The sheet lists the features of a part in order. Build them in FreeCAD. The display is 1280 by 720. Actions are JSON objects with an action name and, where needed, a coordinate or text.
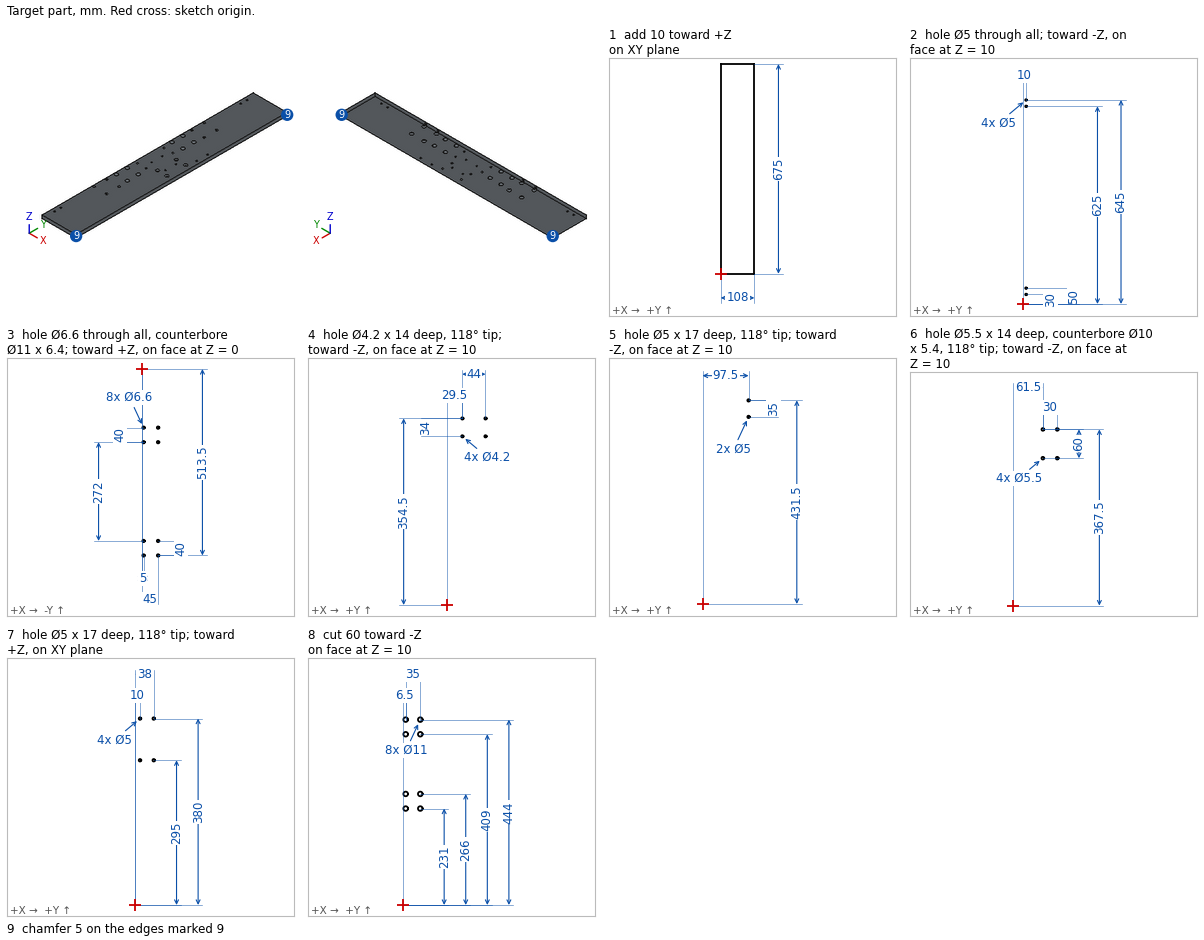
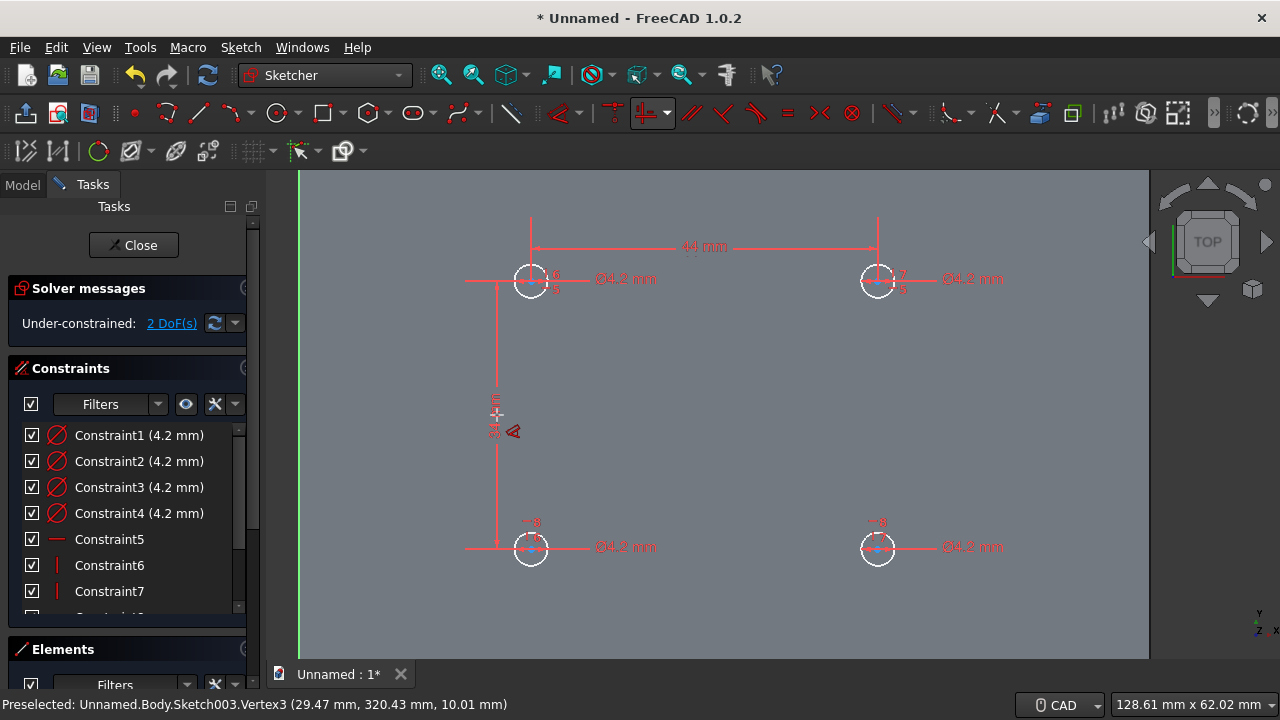
{"action": "left_click", "coordinate": [531, 281]}
{"action": "left_click", "coordinate": [415, 247]}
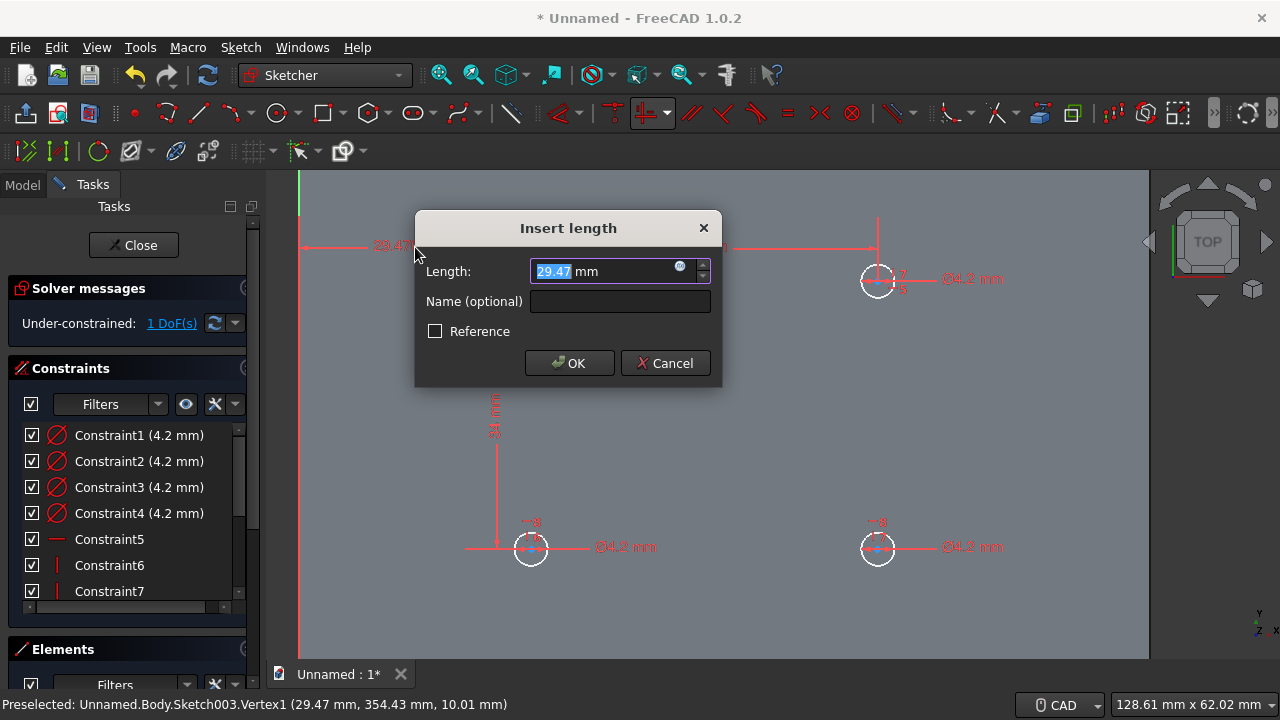
{"action": "type", "text": "29.5"}
{"action": "key", "text": "Return"}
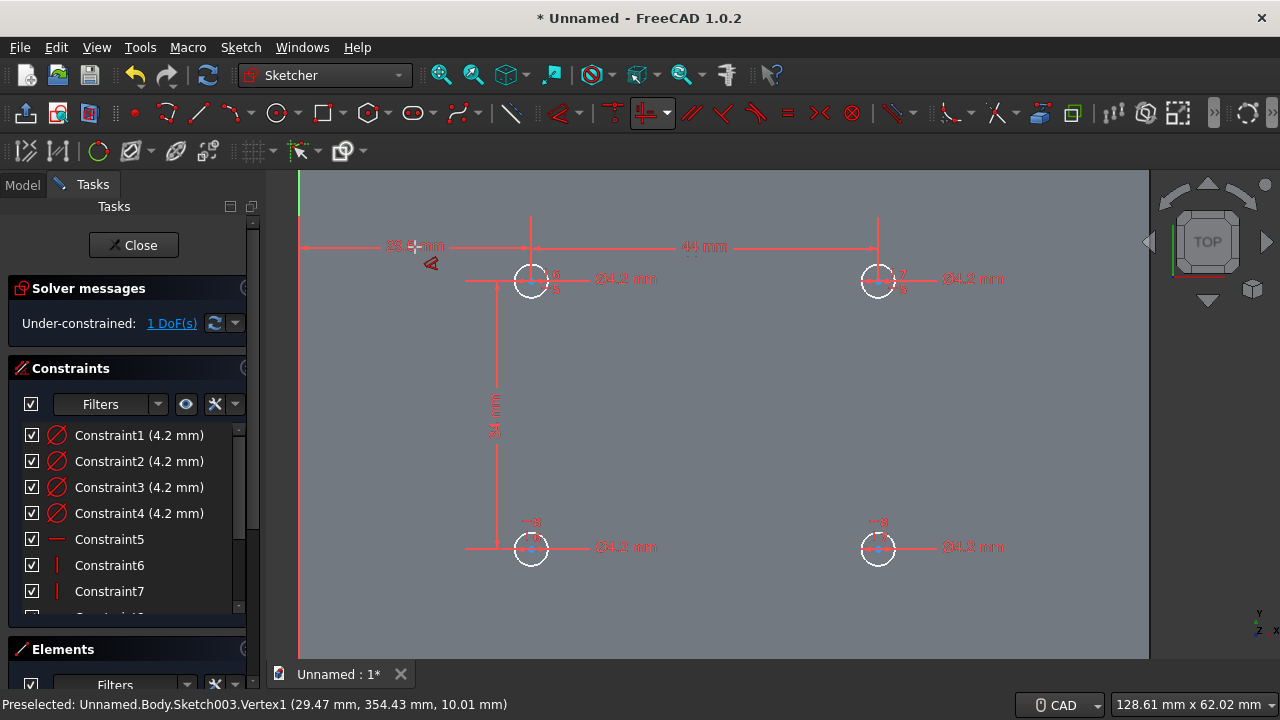
{"action": "left_click", "coordinate": [531, 281]}
{"action": "left_click", "coordinate": [565, 456]}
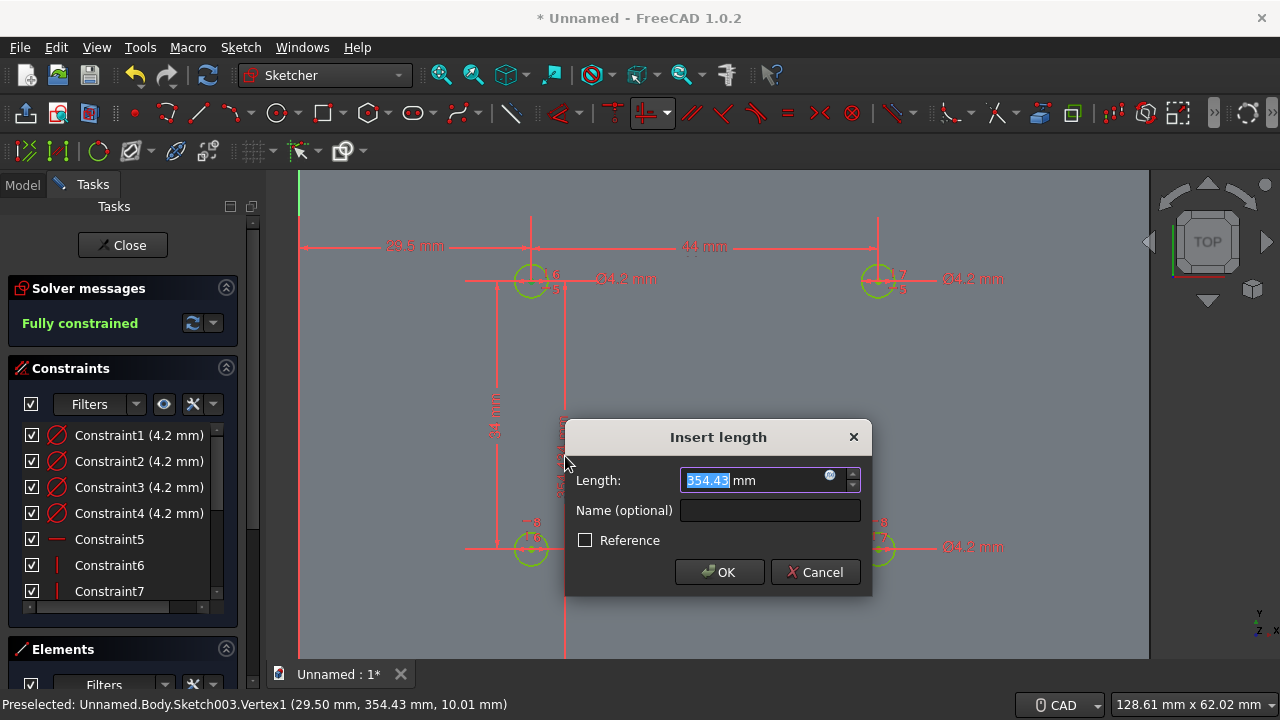
{"action": "type", "text": "354.5"}
{"action": "key", "text": "Return"}
{"action": "key", "text": "Escape"}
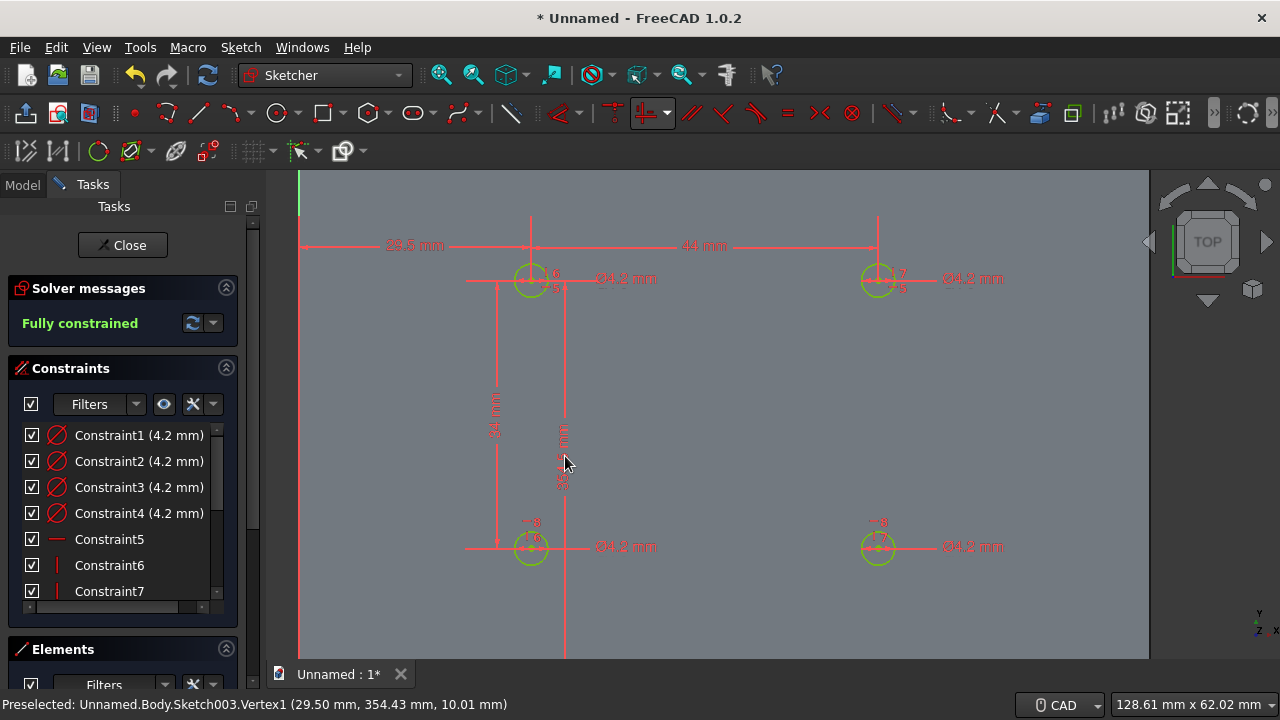
{"action": "left_click", "coordinate": [123, 245]}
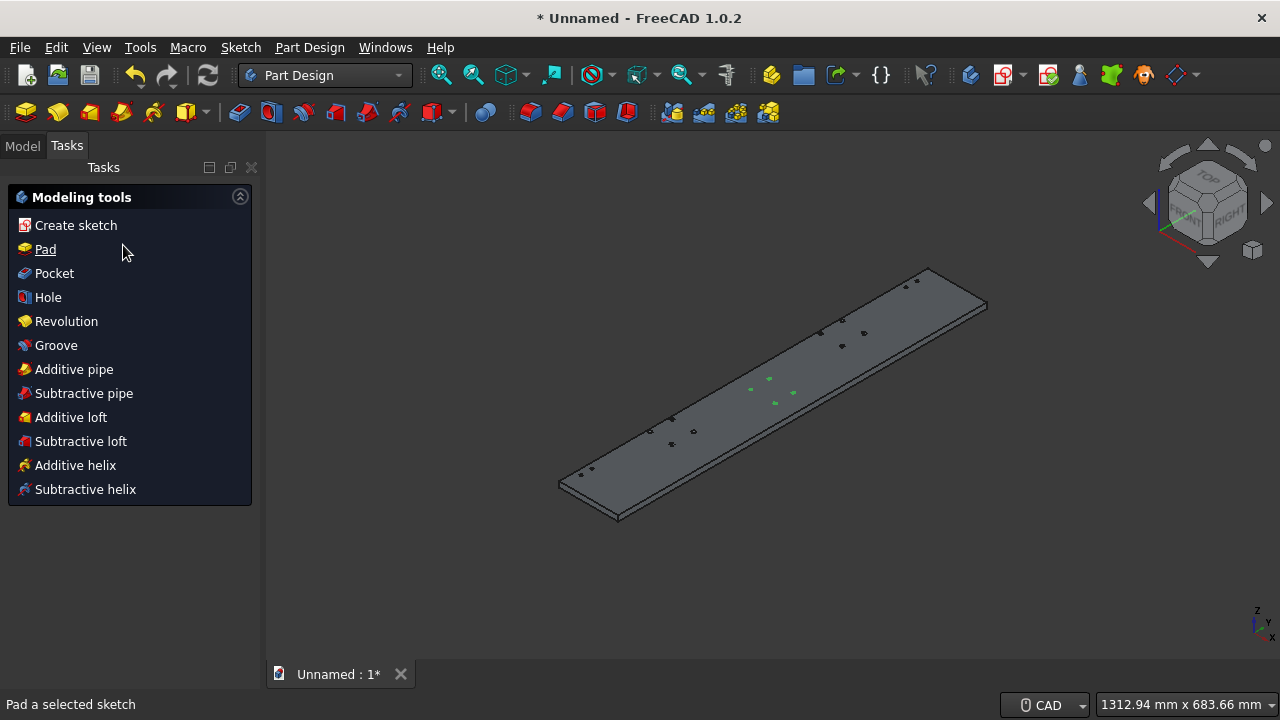
{"action": "left_click", "coordinate": [272, 112]}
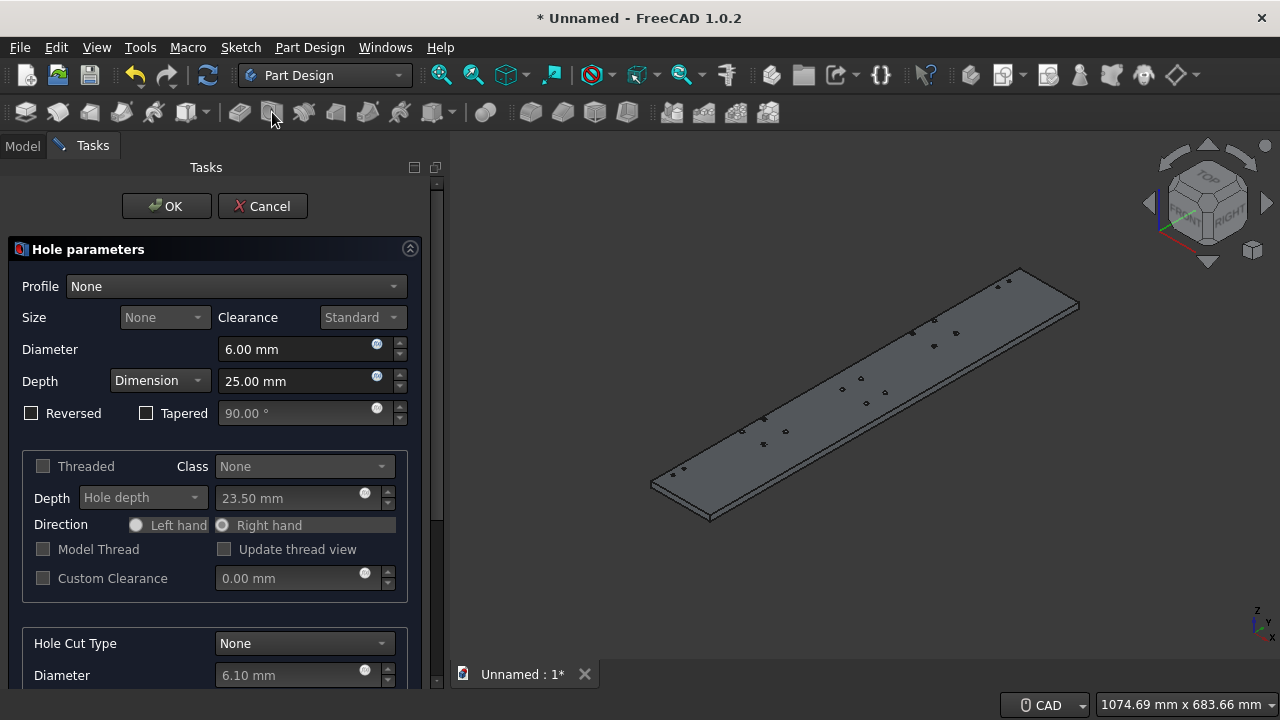
{"action": "triple_click", "coordinate": [305, 349]}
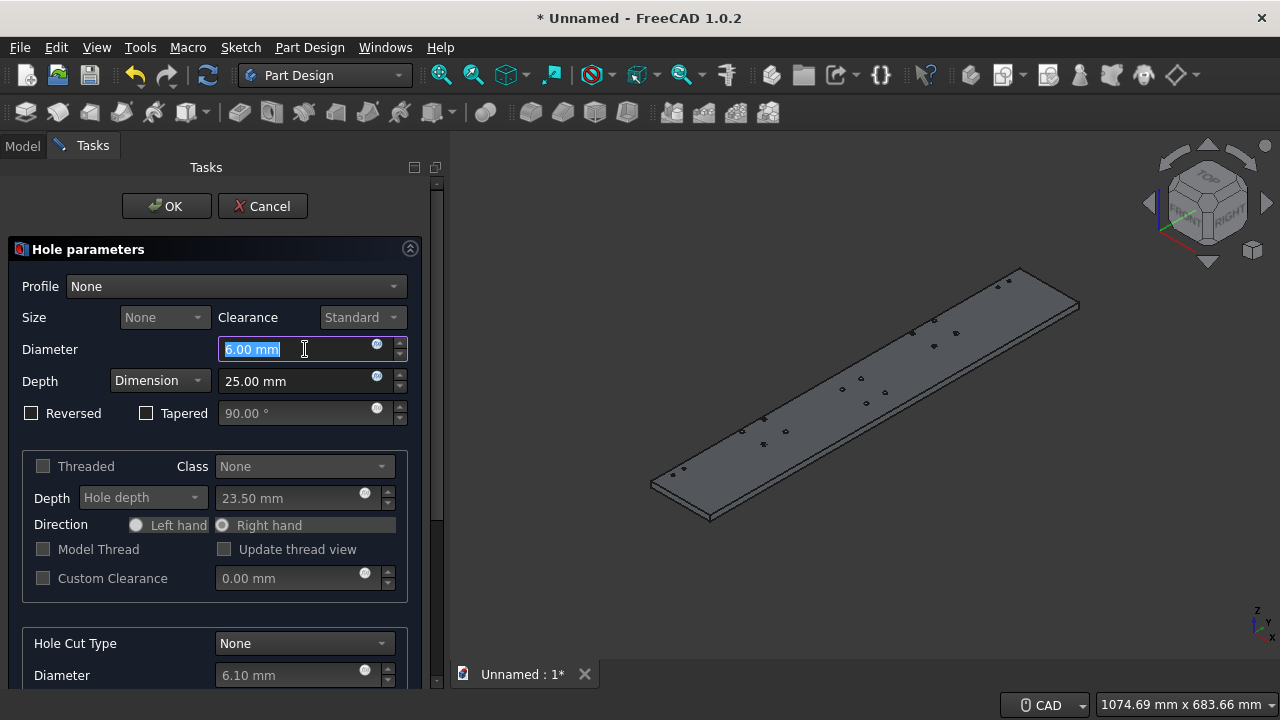
{"action": "type", "text": "4.2"}
{"action": "key", "text": "Tab"}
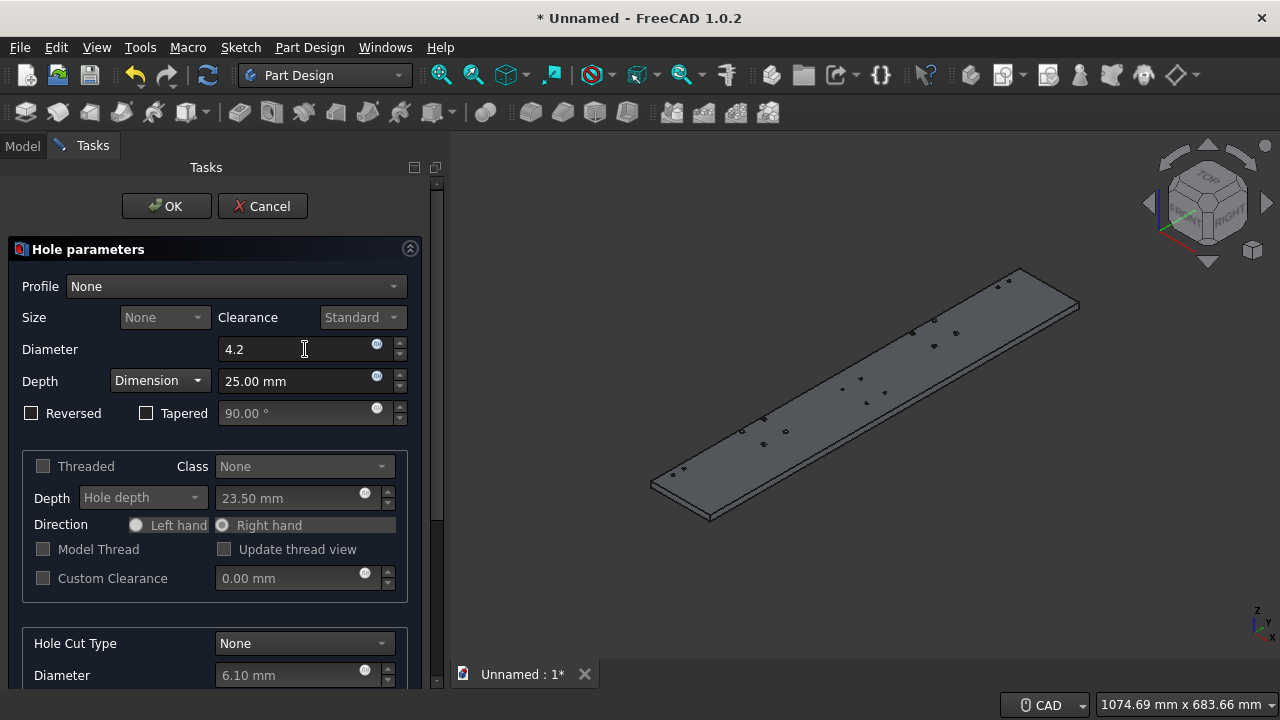
{"action": "triple_click", "coordinate": [305, 381]}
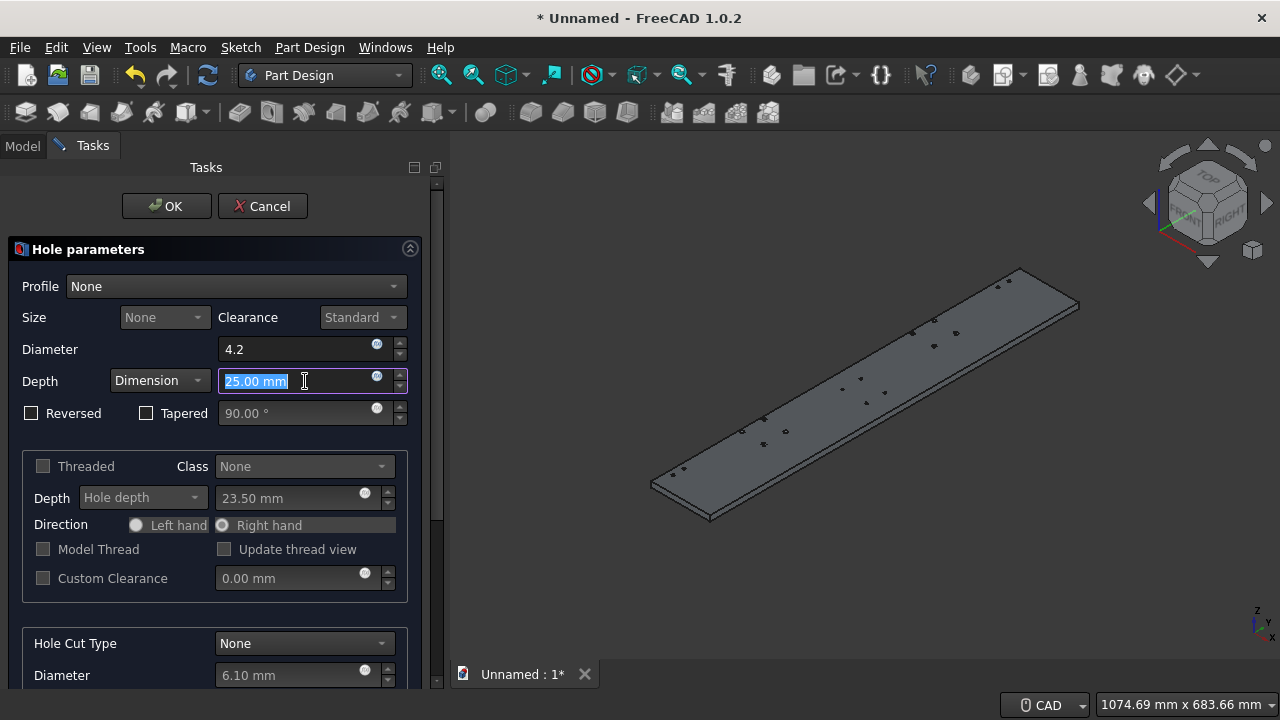
{"action": "type", "text": "14"}
{"action": "key", "text": "Tab"}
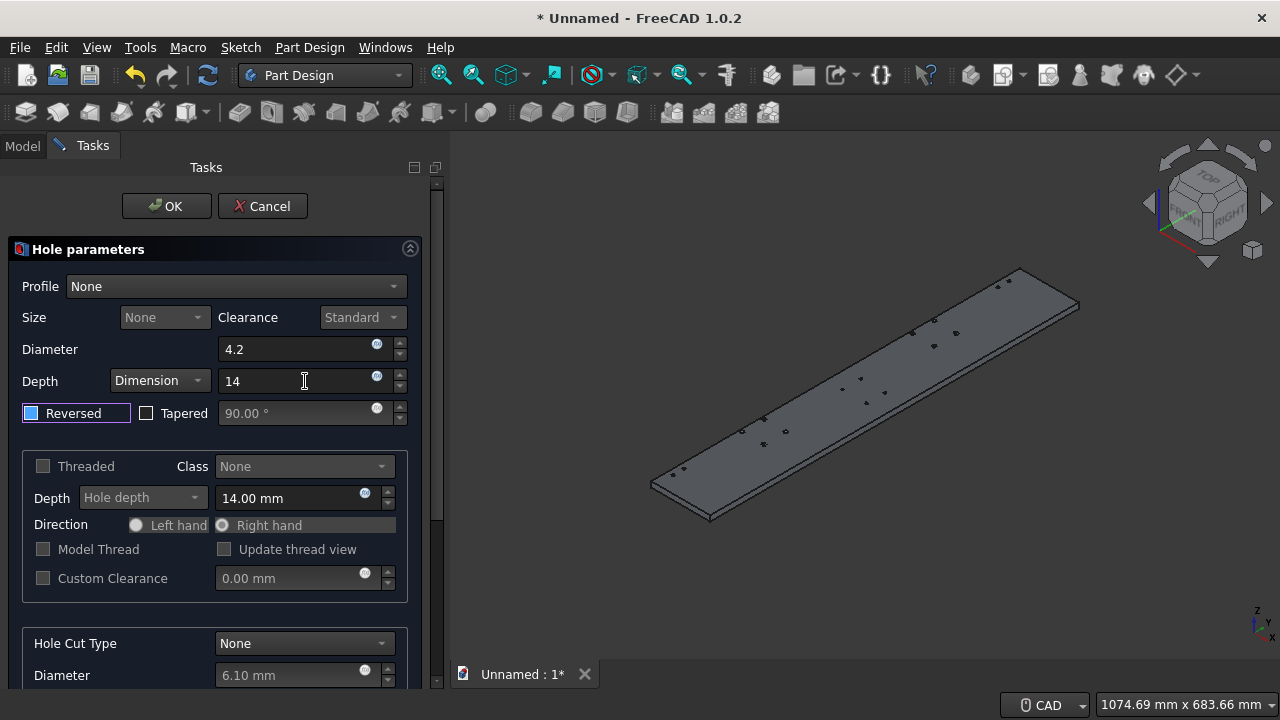
{"action": "left_click", "coordinate": [167, 206]}